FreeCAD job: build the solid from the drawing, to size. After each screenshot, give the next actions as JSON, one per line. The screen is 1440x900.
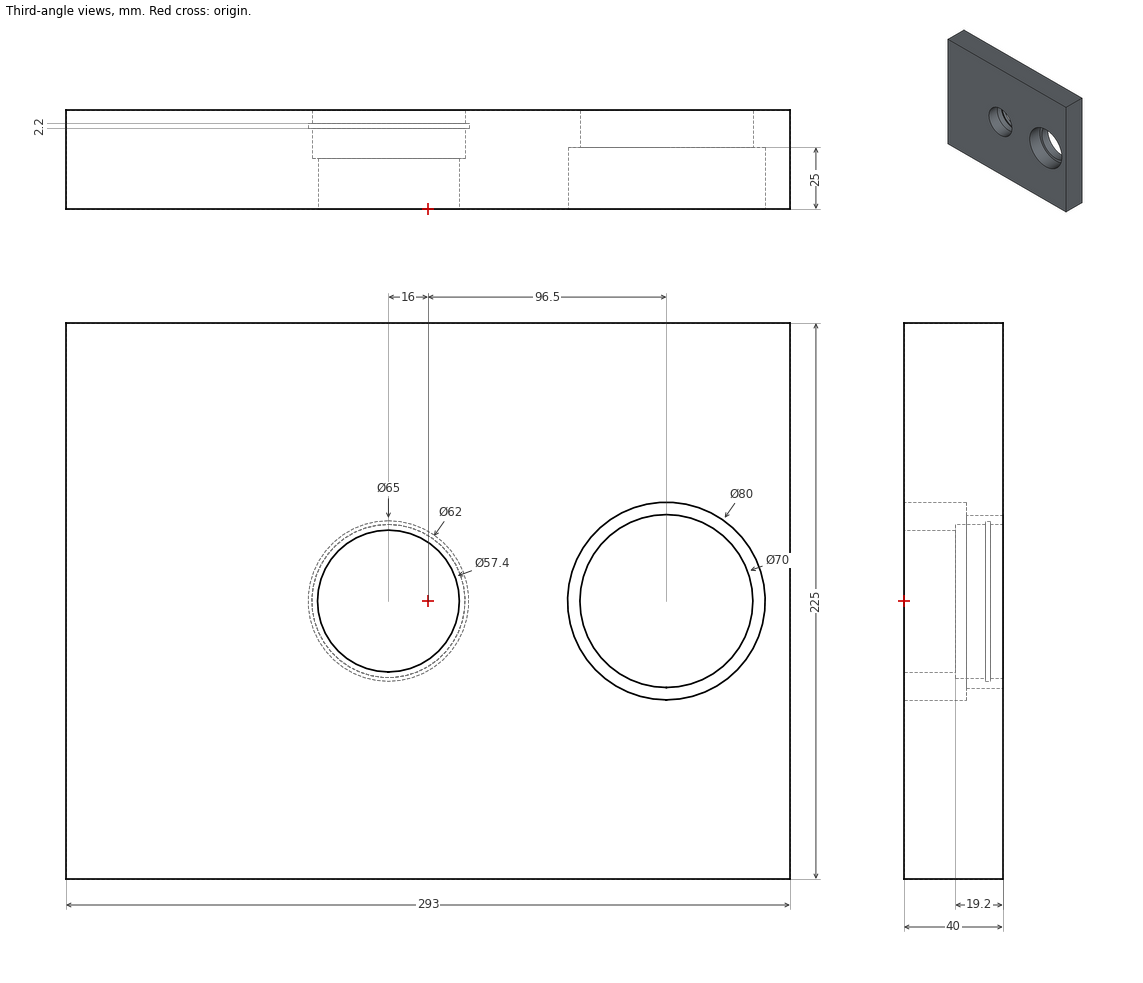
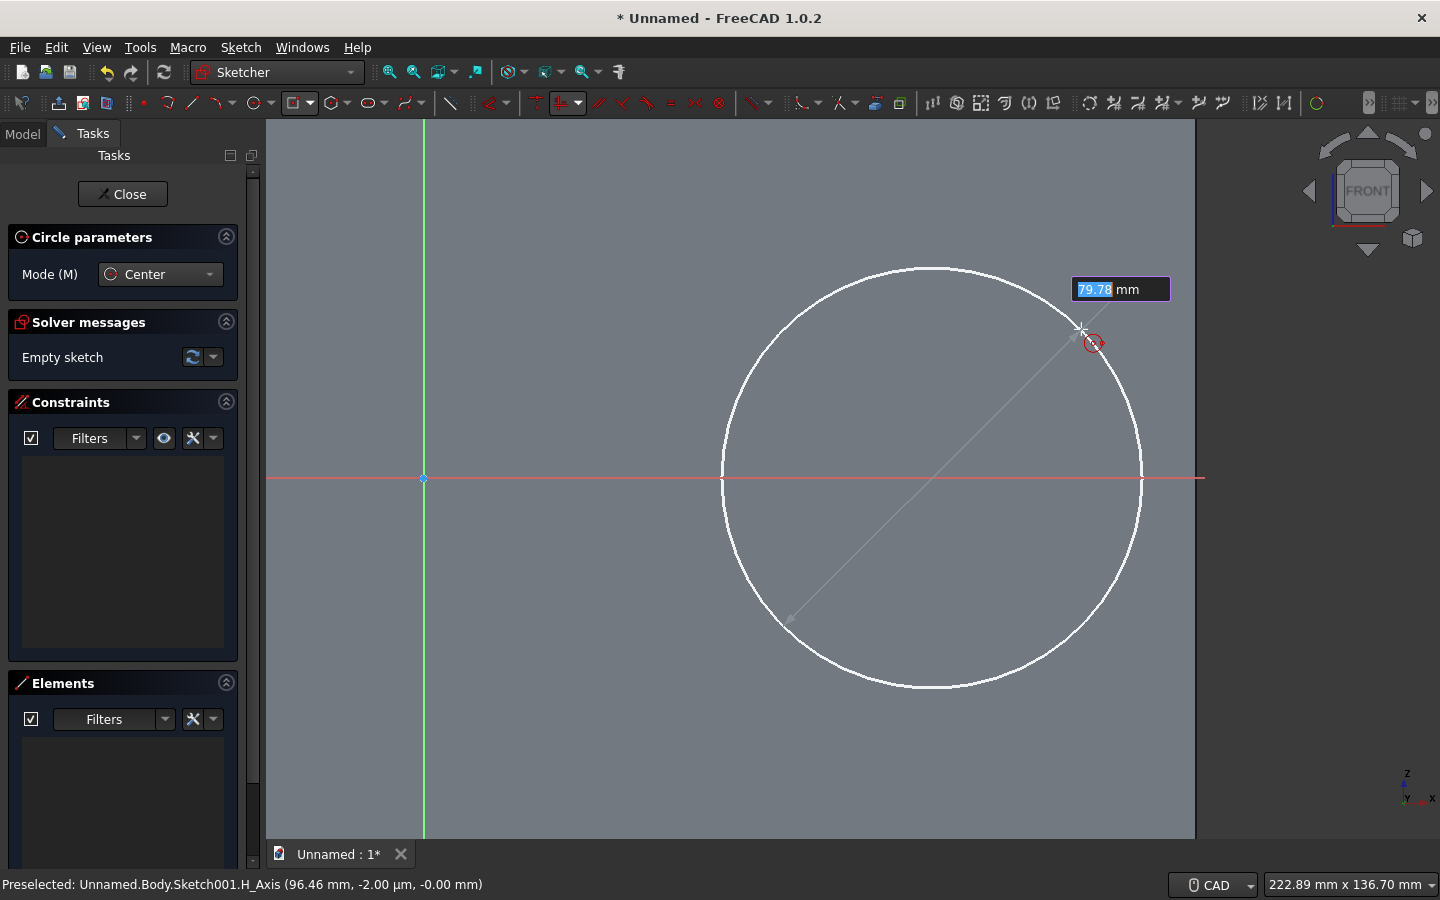
{"action": "type", "text": "80"}
{"action": "key", "text": "Return"}
{"action": "key", "text": "Escape"}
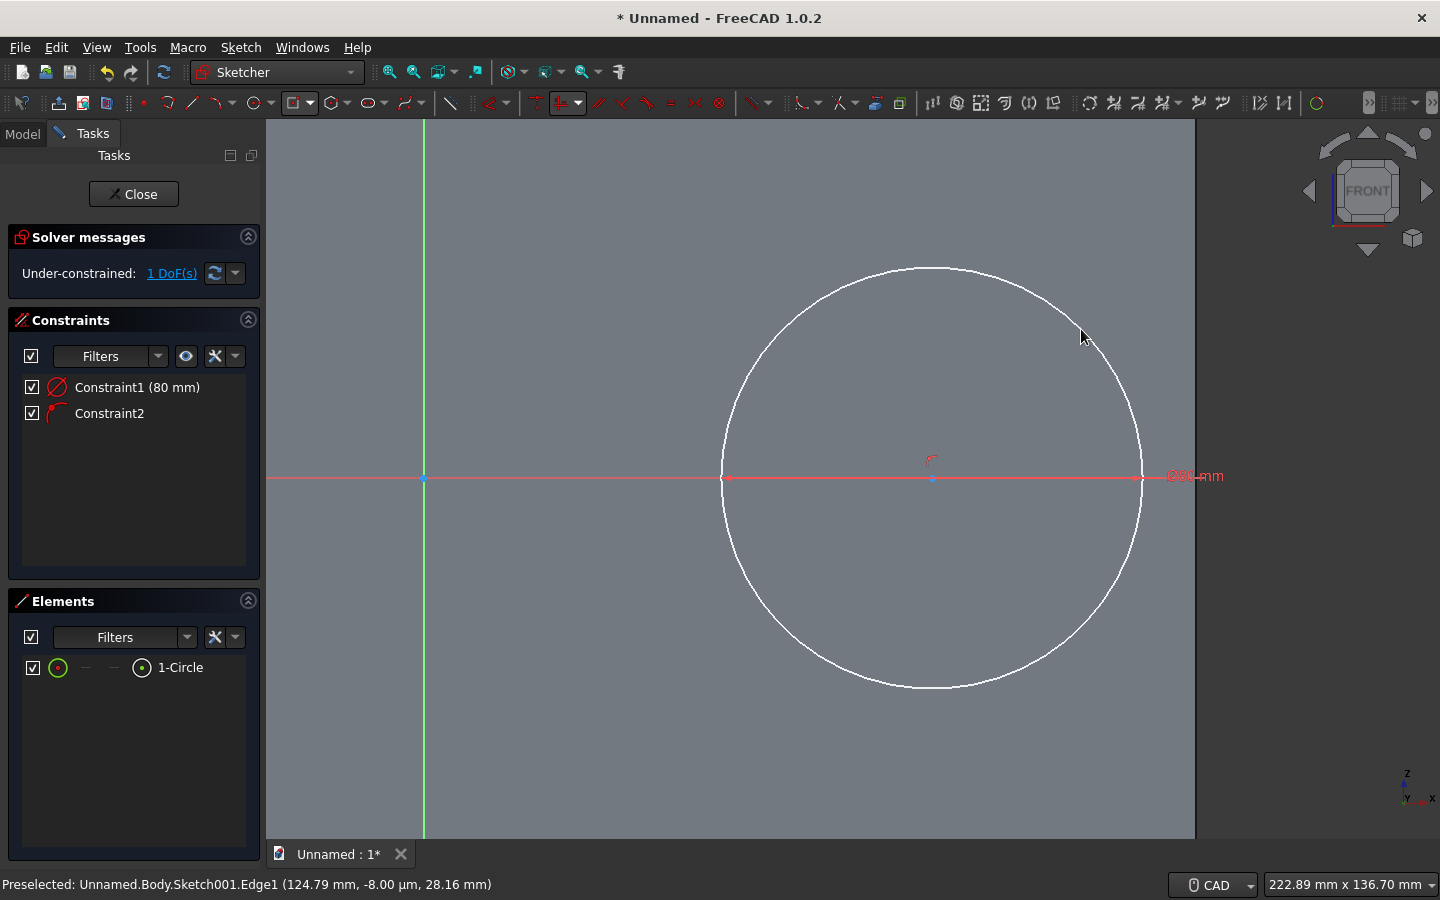
{"action": "left_click", "coordinate": [490, 104]}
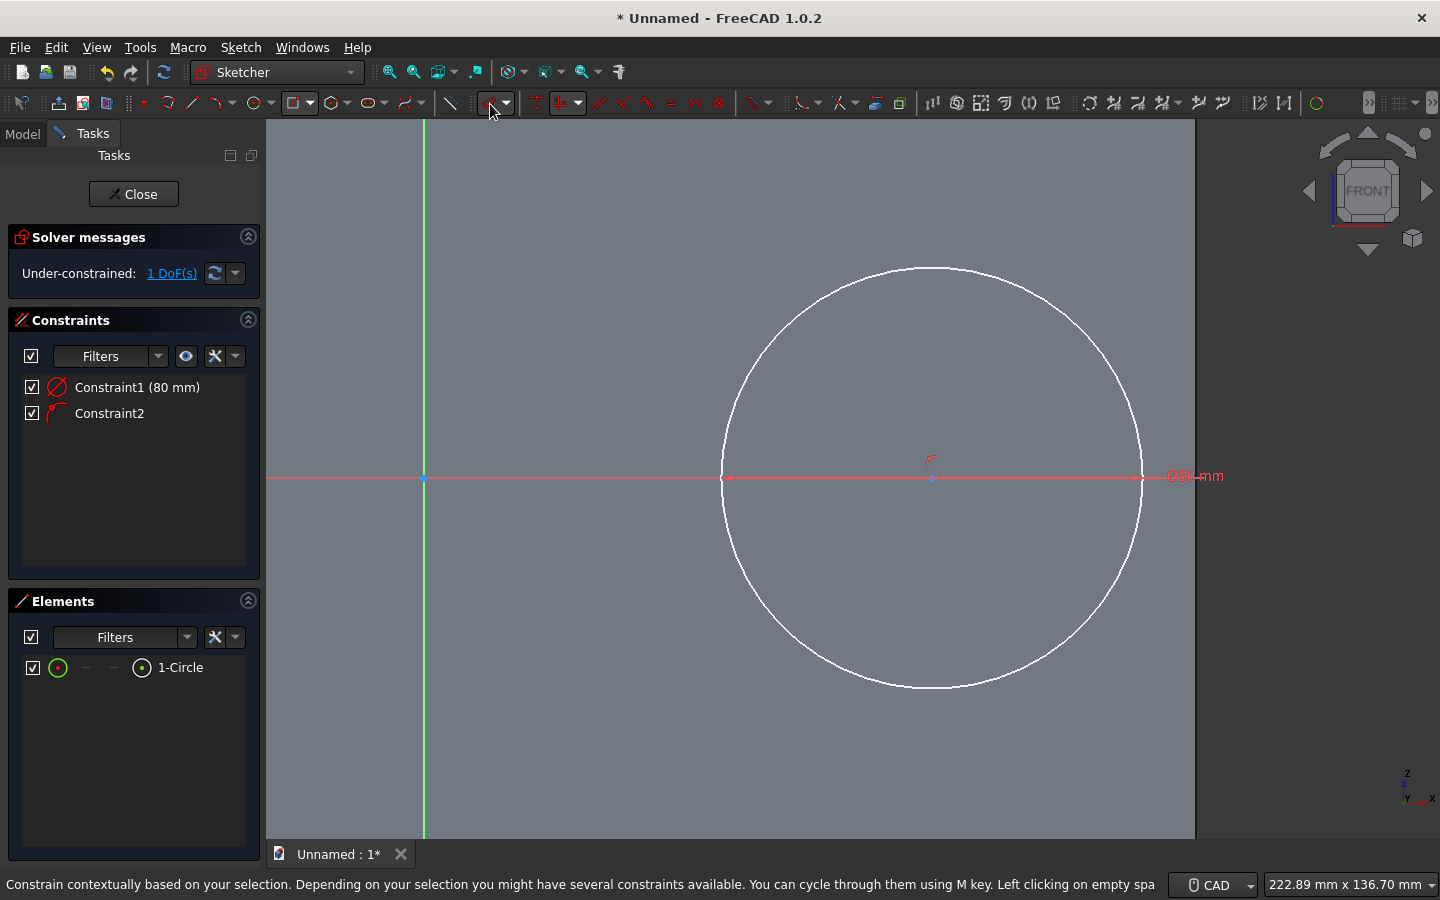
{"action": "left_click", "coordinate": [932, 478]}
{"action": "left_click", "coordinate": [678, 512]}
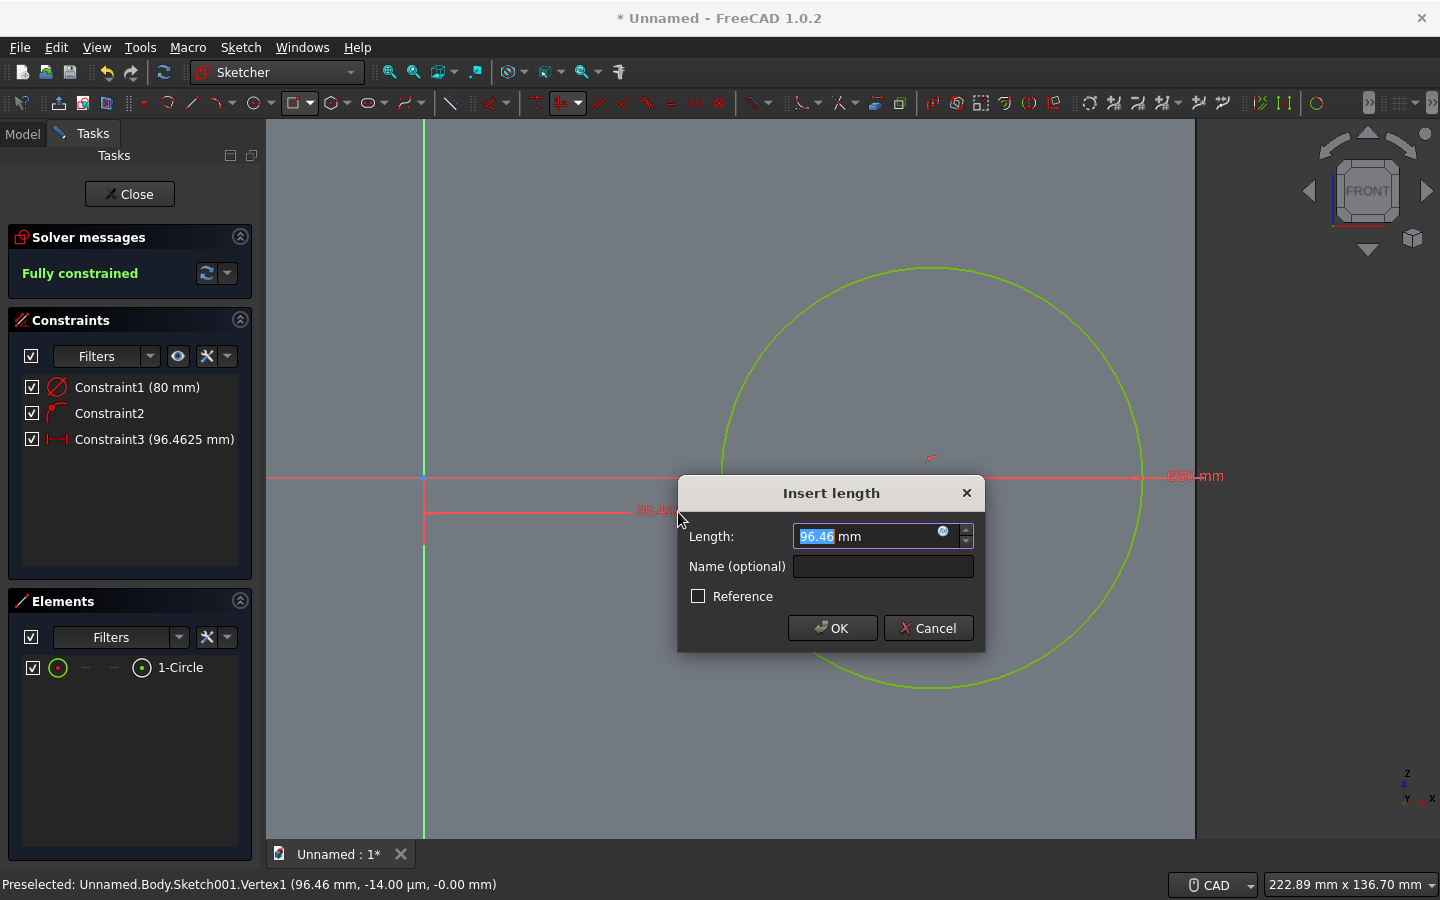
{"action": "type", "text": "96.5"}
{"action": "key", "text": "Return"}
{"action": "key", "text": "Escape"}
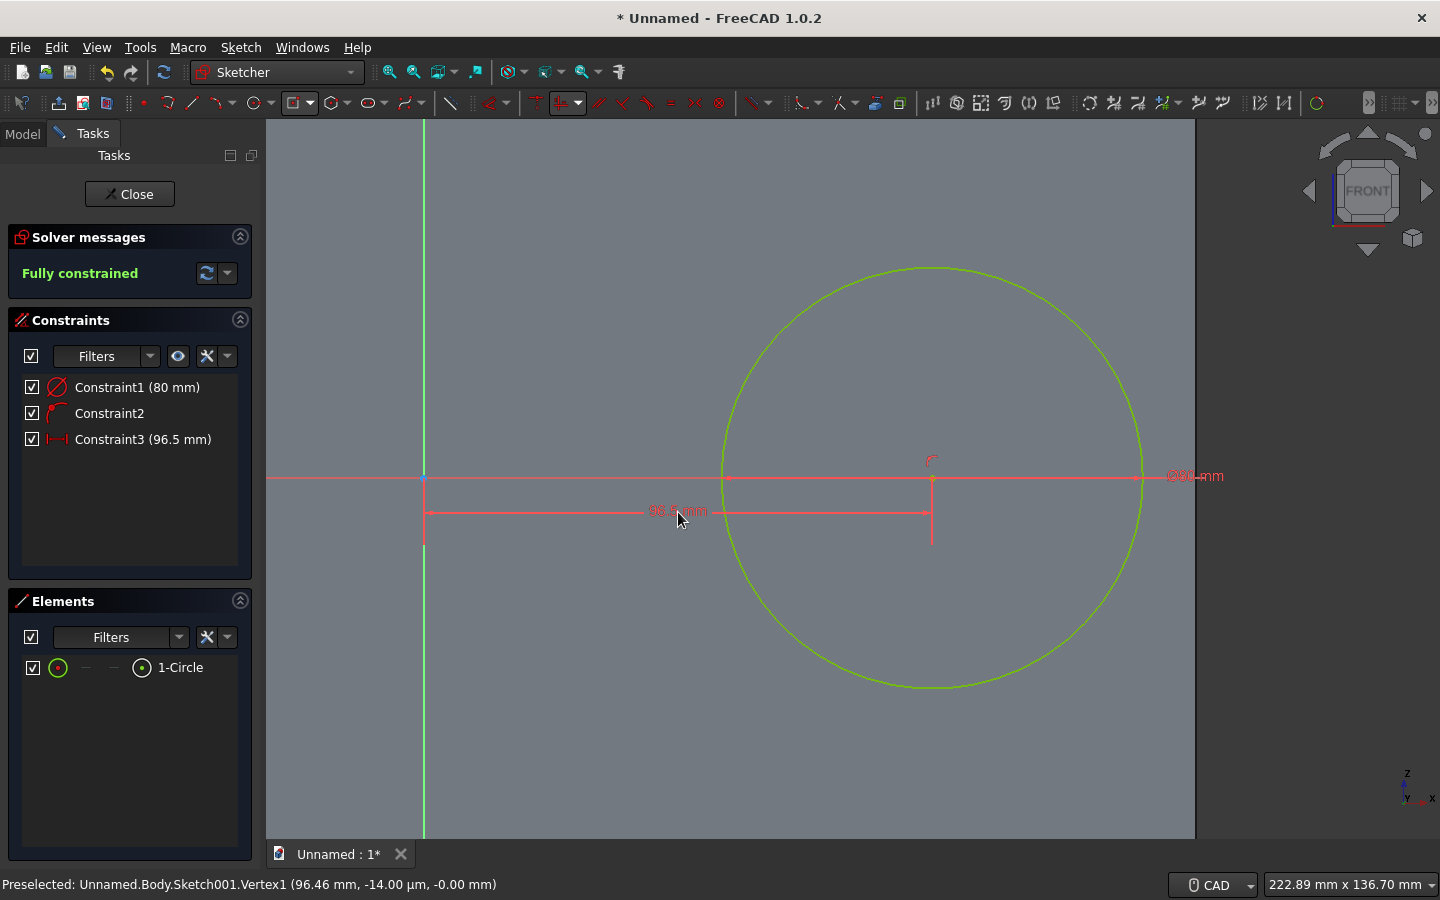
{"action": "left_click", "coordinate": [130, 194]}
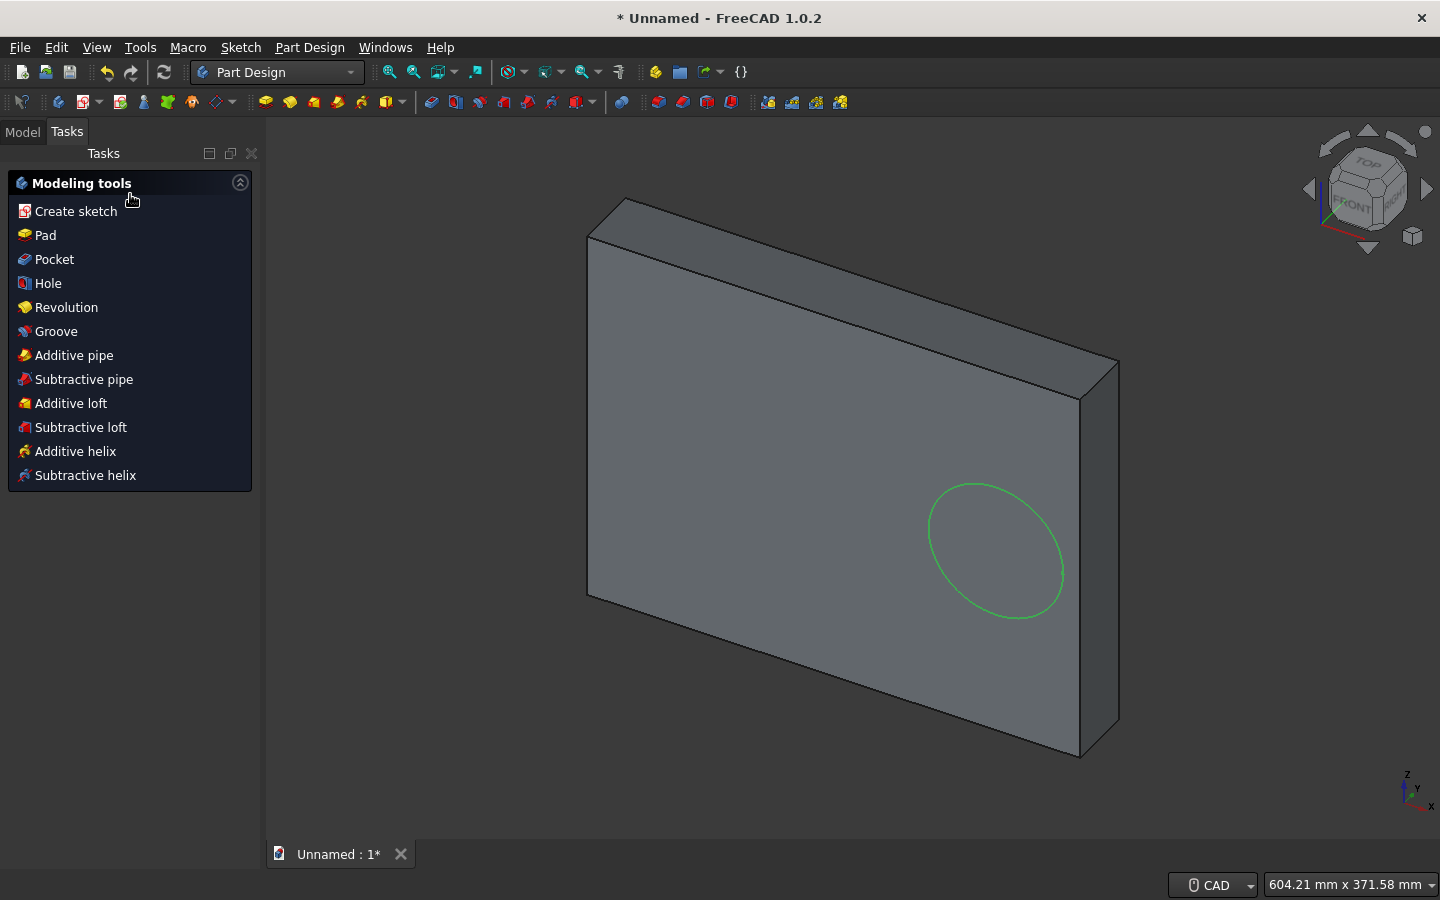
{"action": "left_click", "coordinate": [432, 102]}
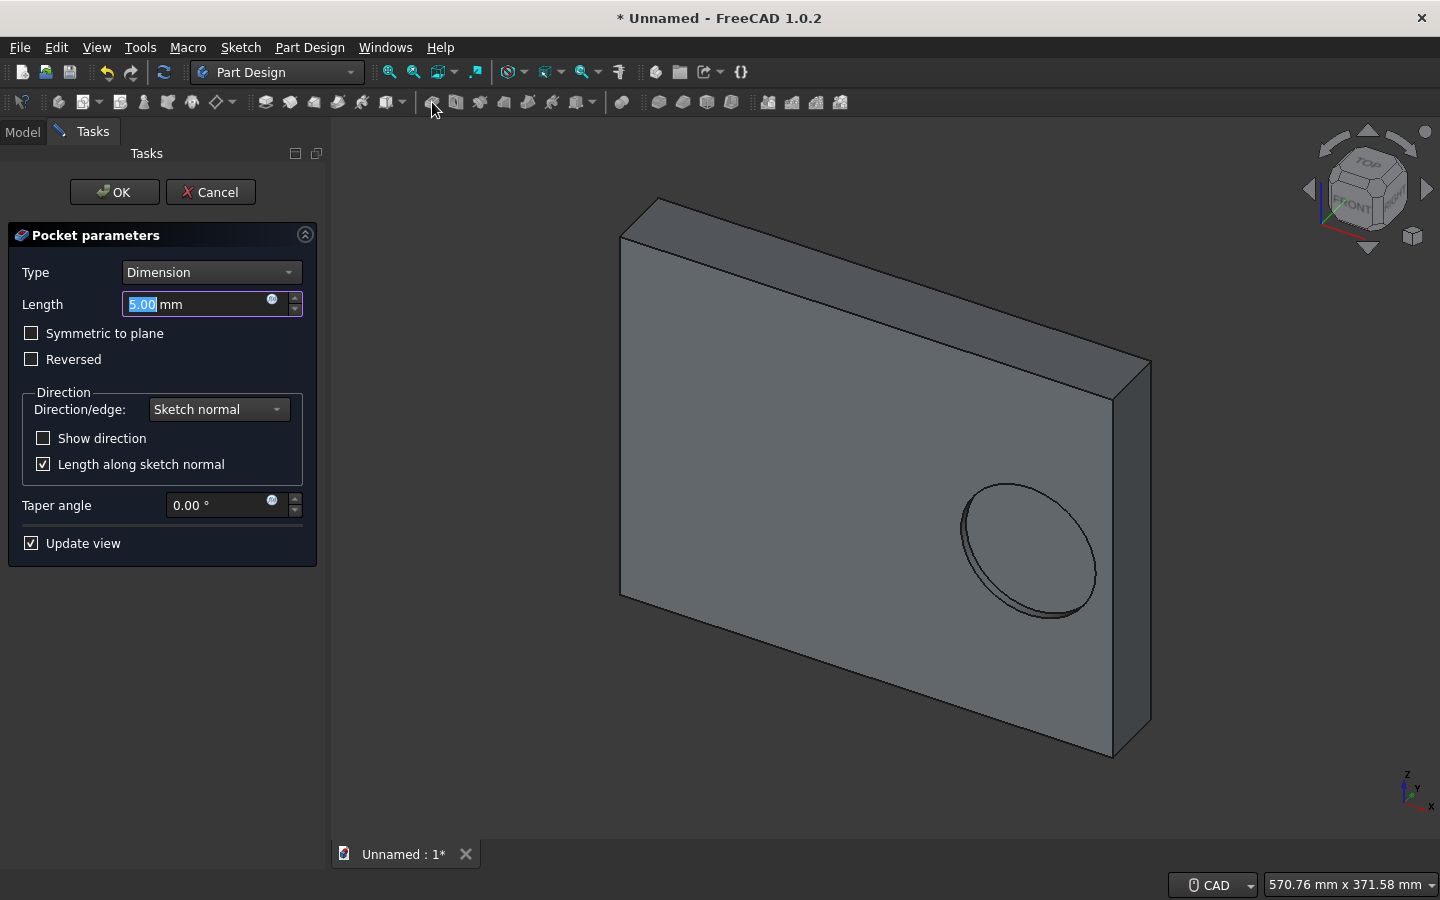
{"action": "type", "text": "25"}
{"action": "key", "text": "Tab"}